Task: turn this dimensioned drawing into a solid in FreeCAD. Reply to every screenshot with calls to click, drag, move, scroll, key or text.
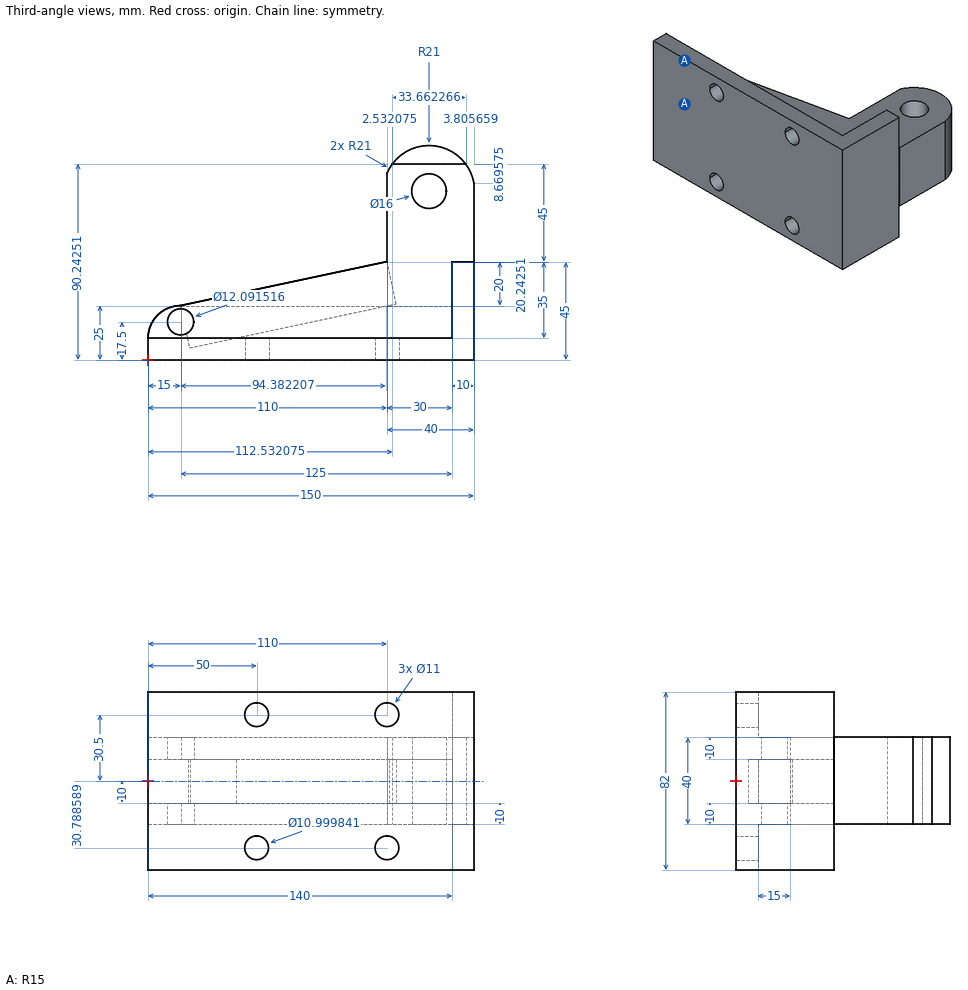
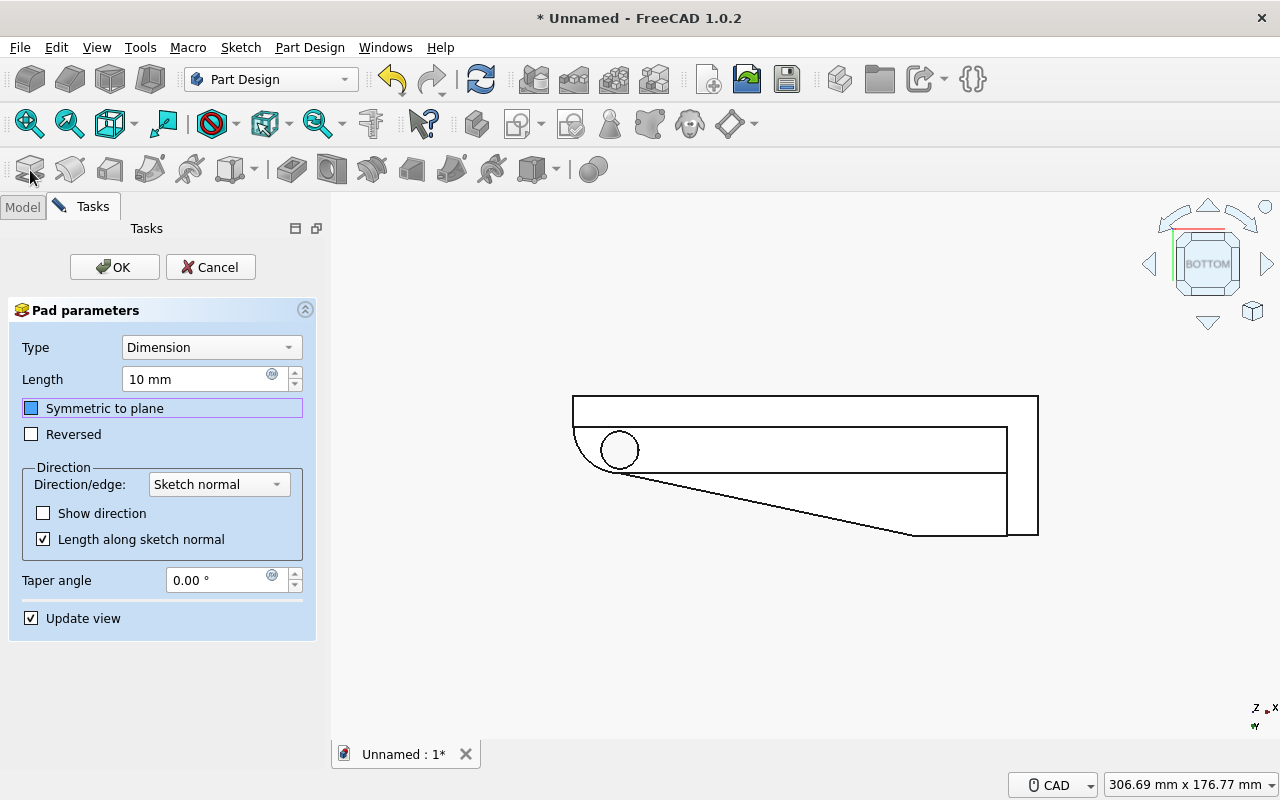
click(30, 434)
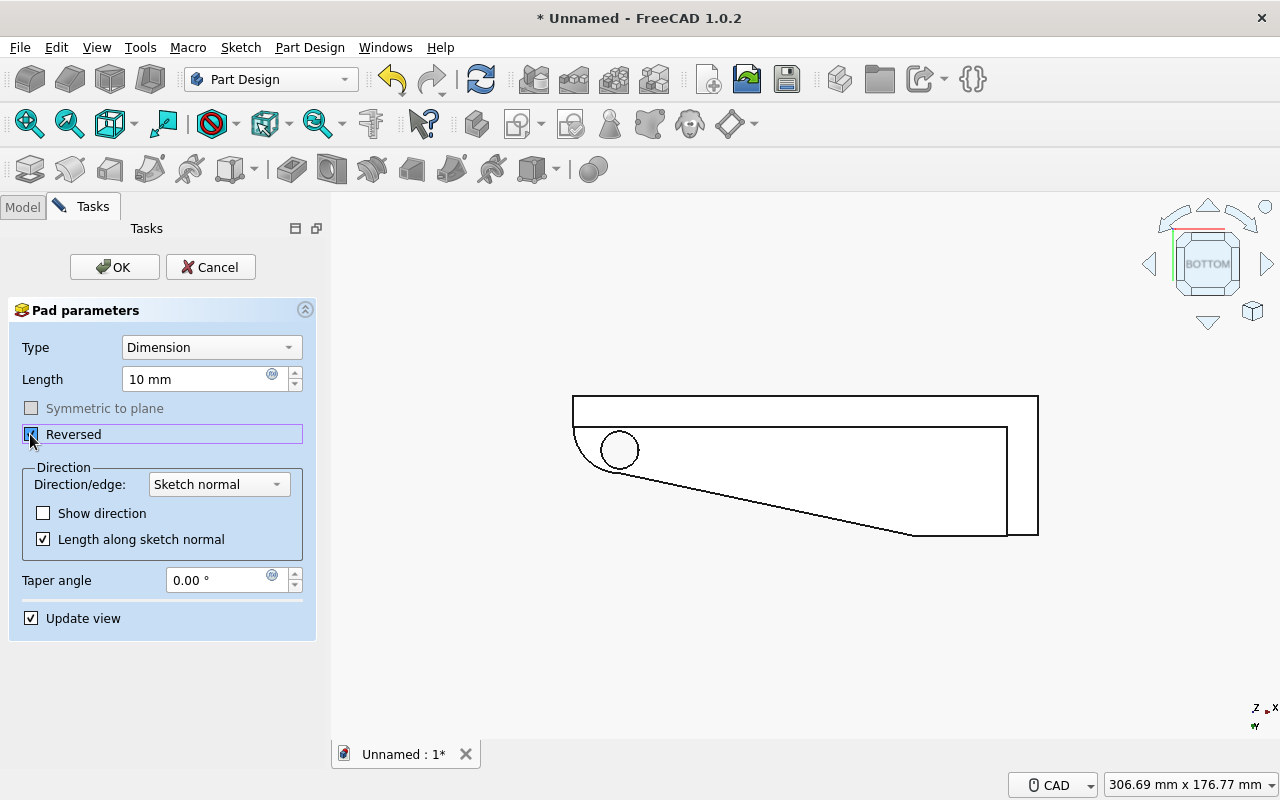
click(115, 267)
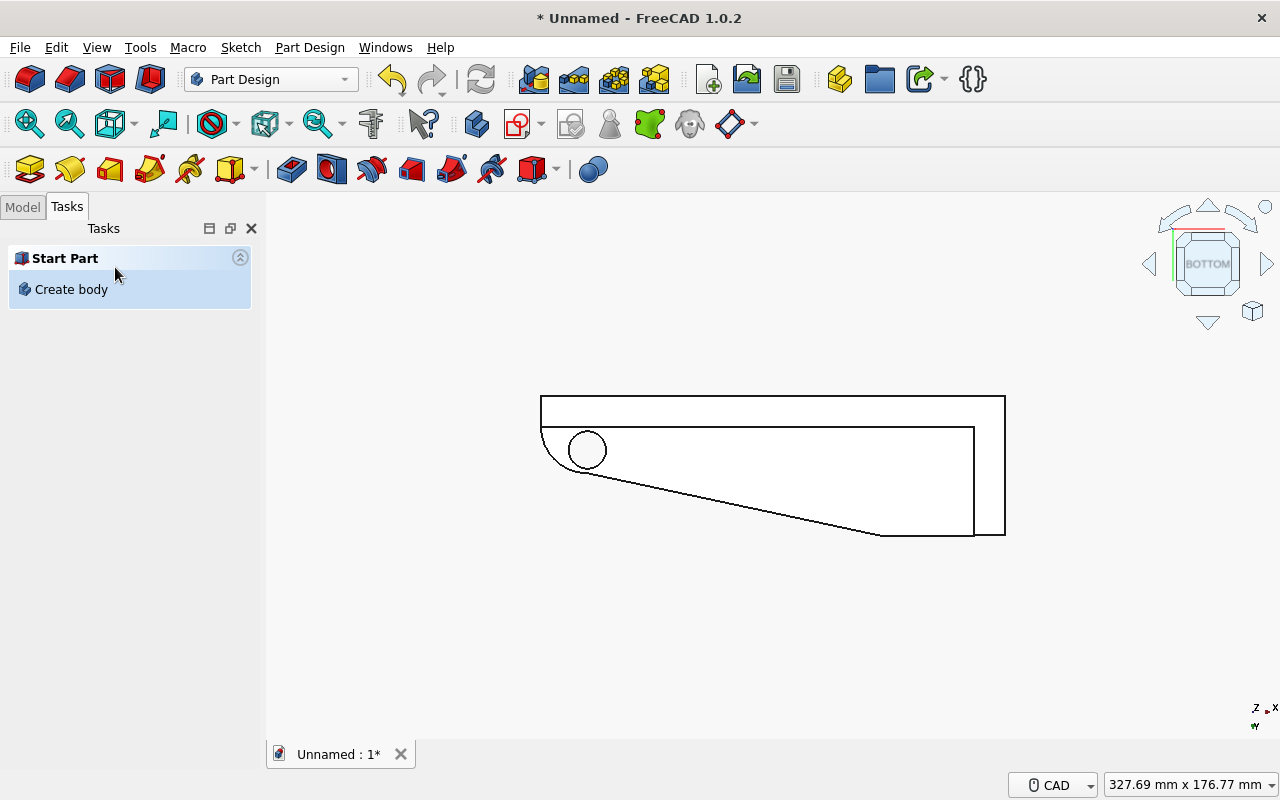
click(881, 480)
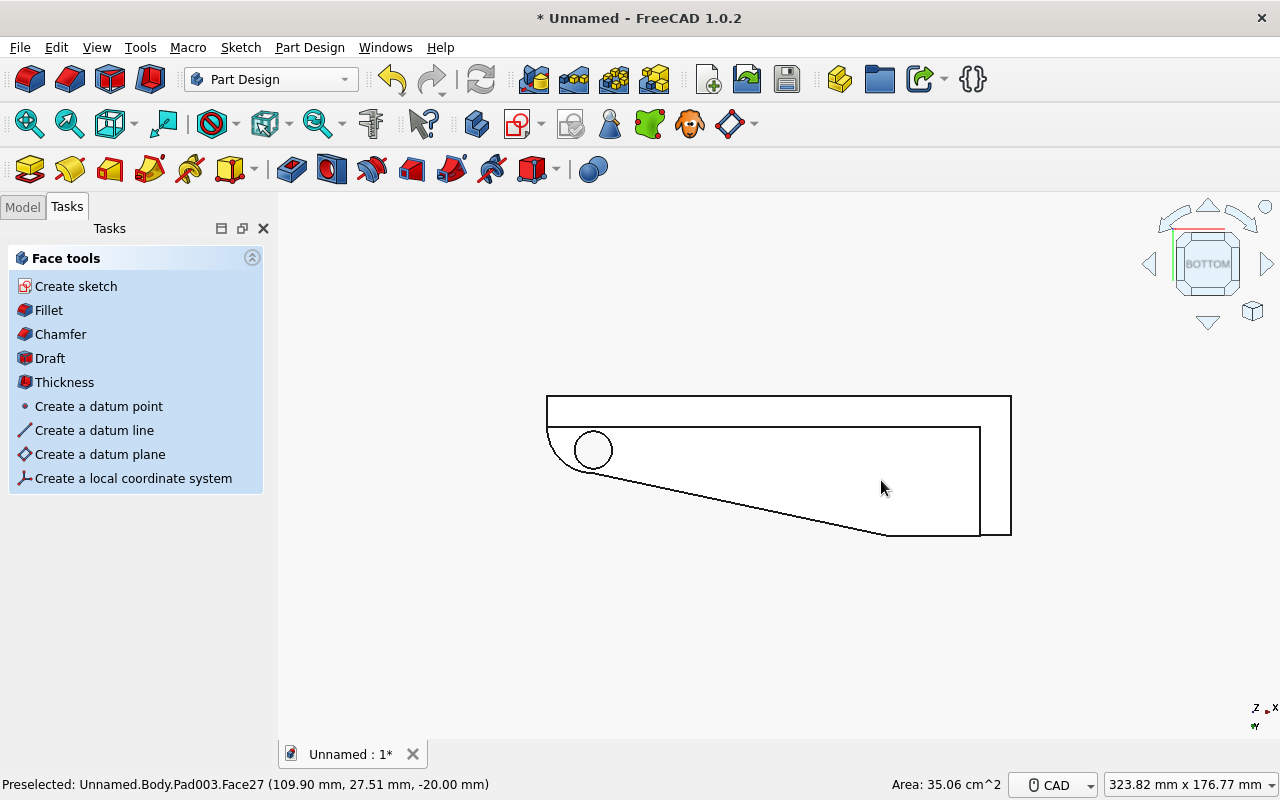
click(518, 124)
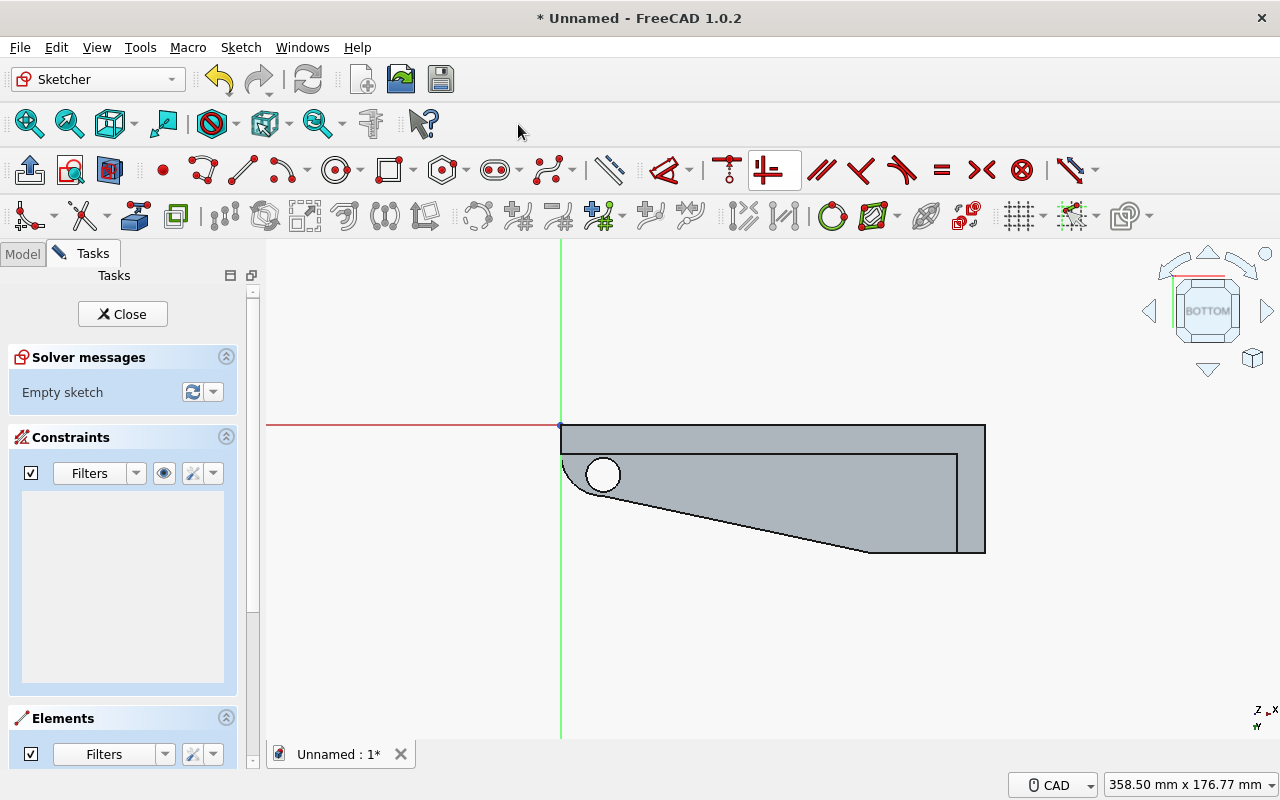
key(q)
key(s)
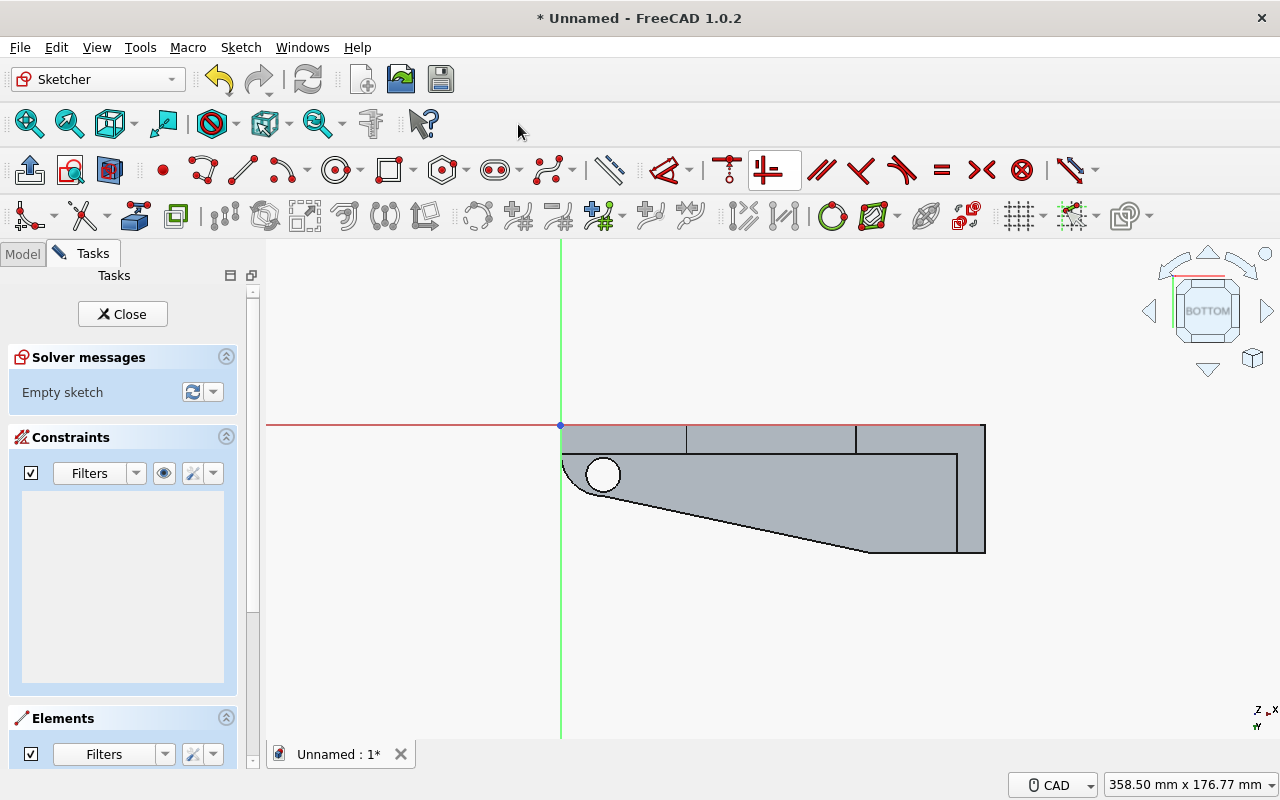
scroll(869, 490, up, 2)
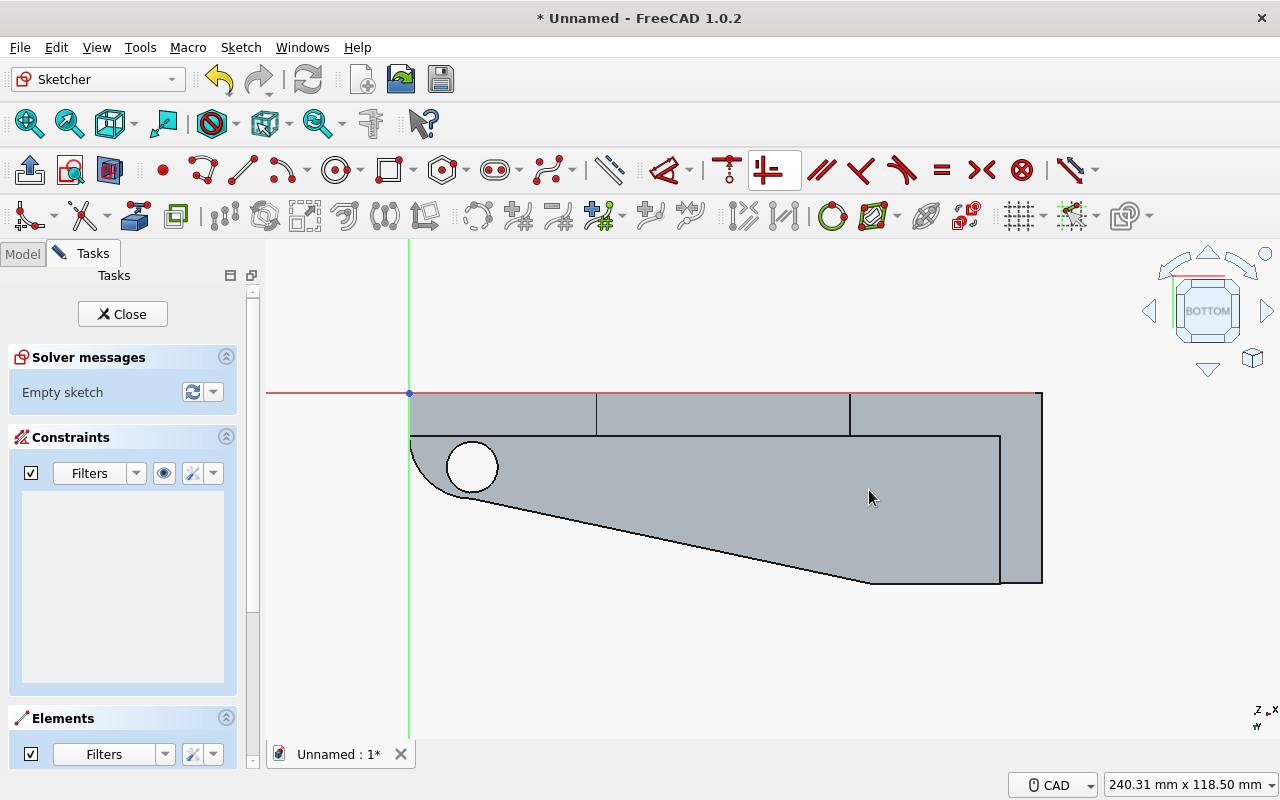
key(g)
key(m)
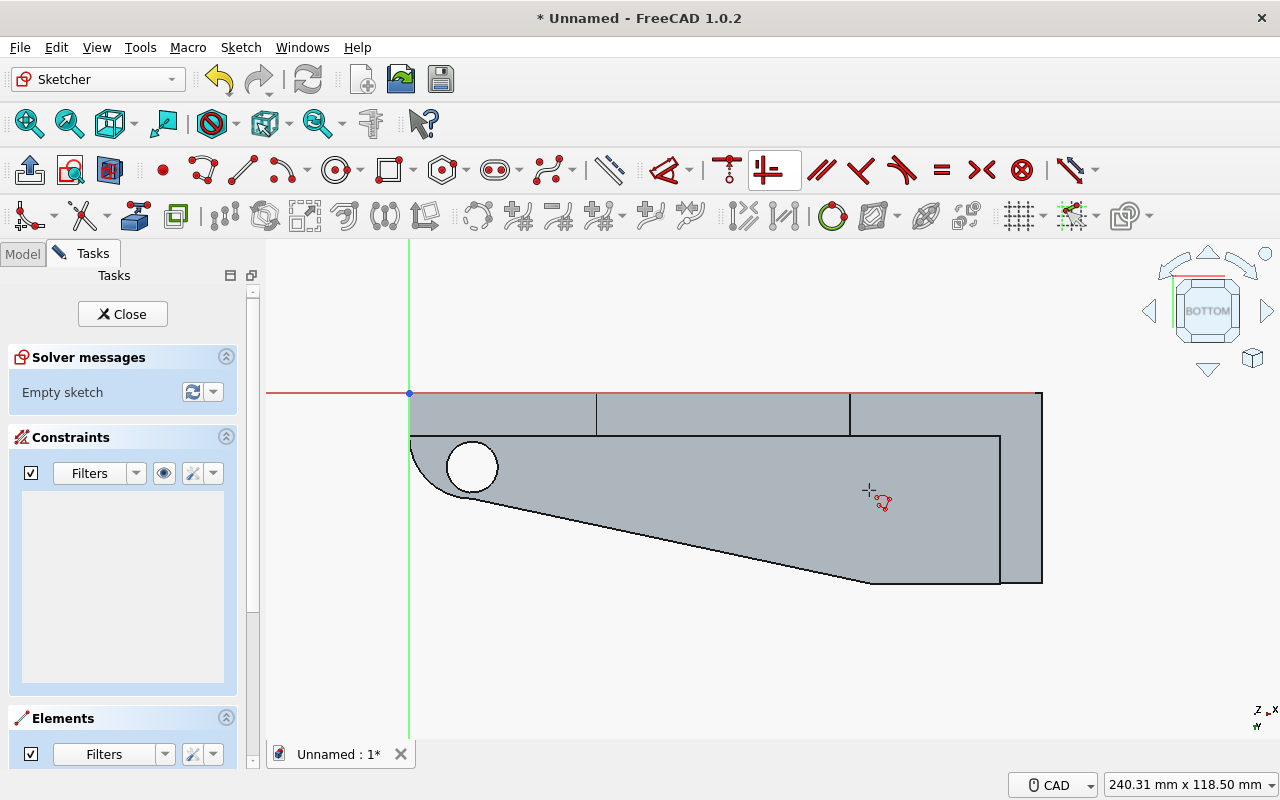
click(472, 499)
click(873, 584)
click(1000, 584)
click(1000, 499)
click(472, 500)
key(Escape)
key(Escape)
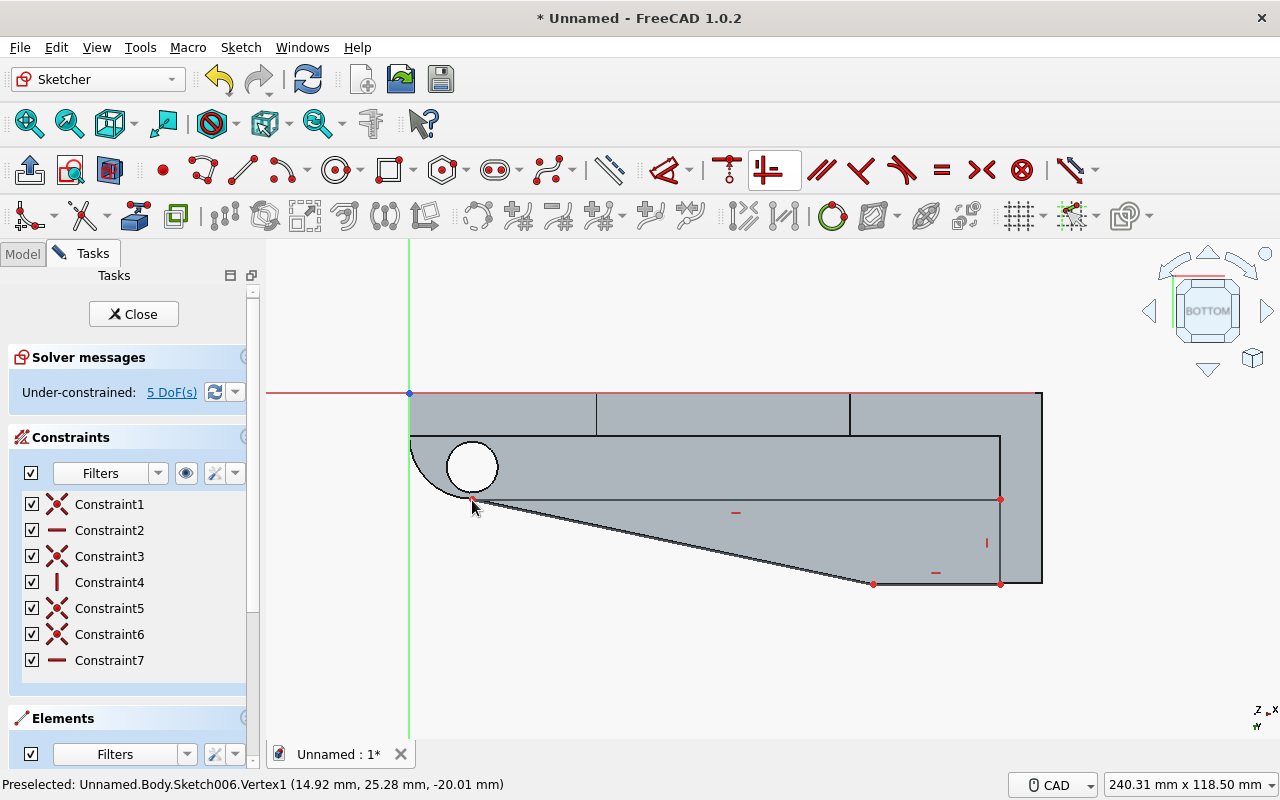
click(664, 170)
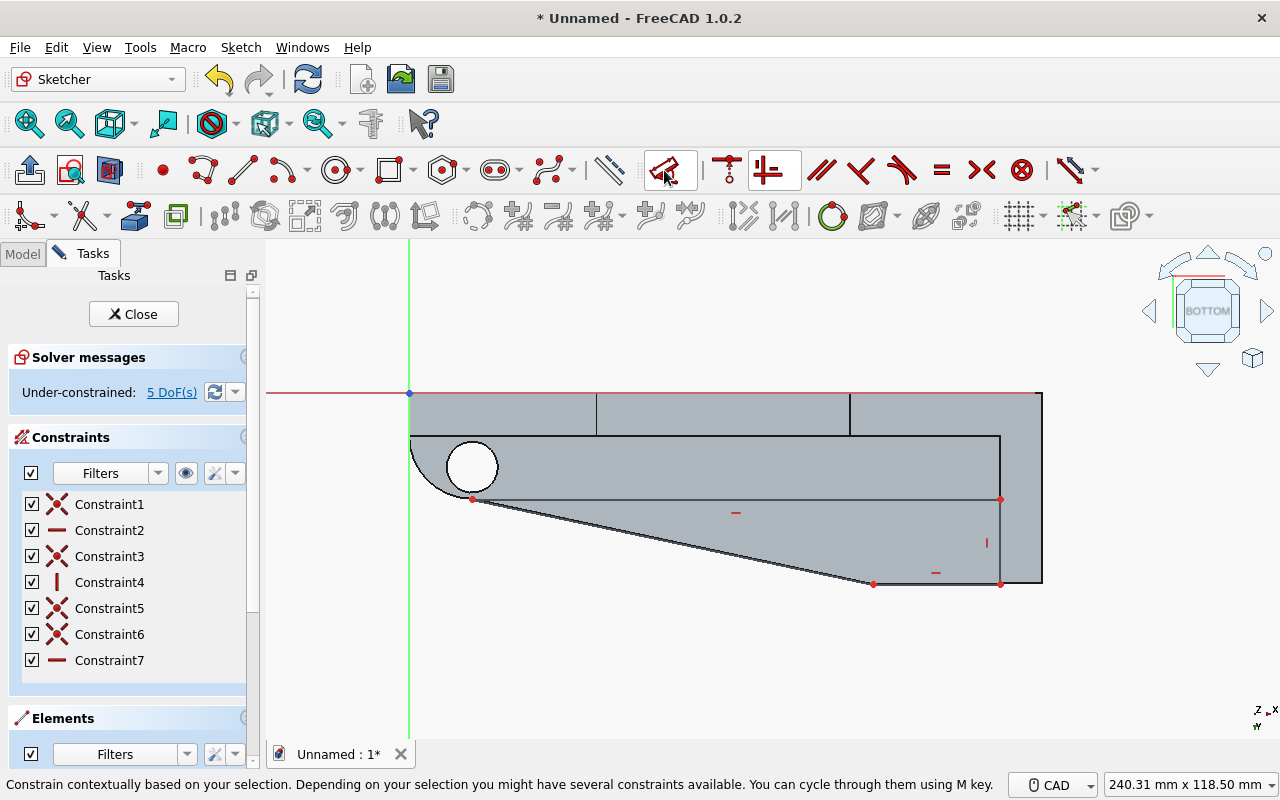
click(911, 585)
click(937, 619)